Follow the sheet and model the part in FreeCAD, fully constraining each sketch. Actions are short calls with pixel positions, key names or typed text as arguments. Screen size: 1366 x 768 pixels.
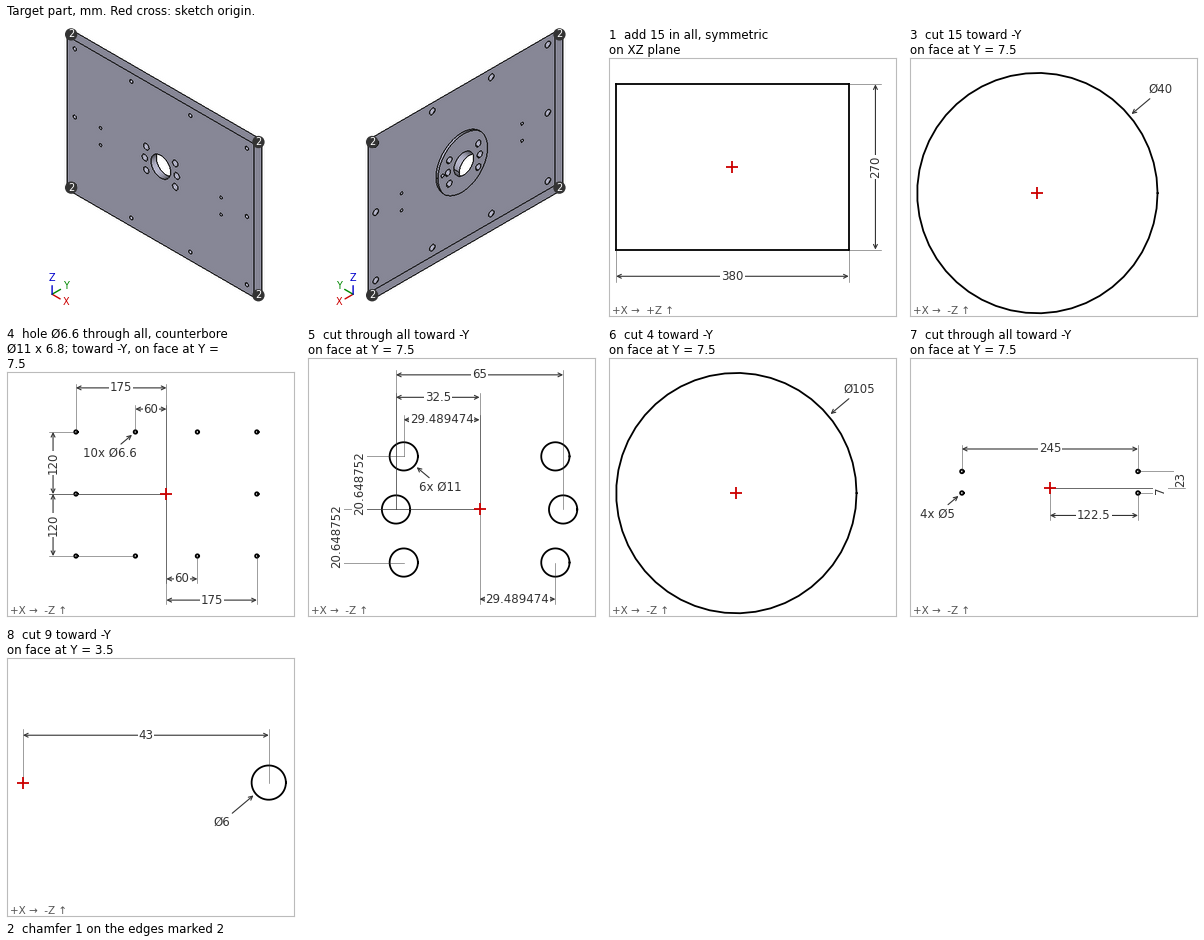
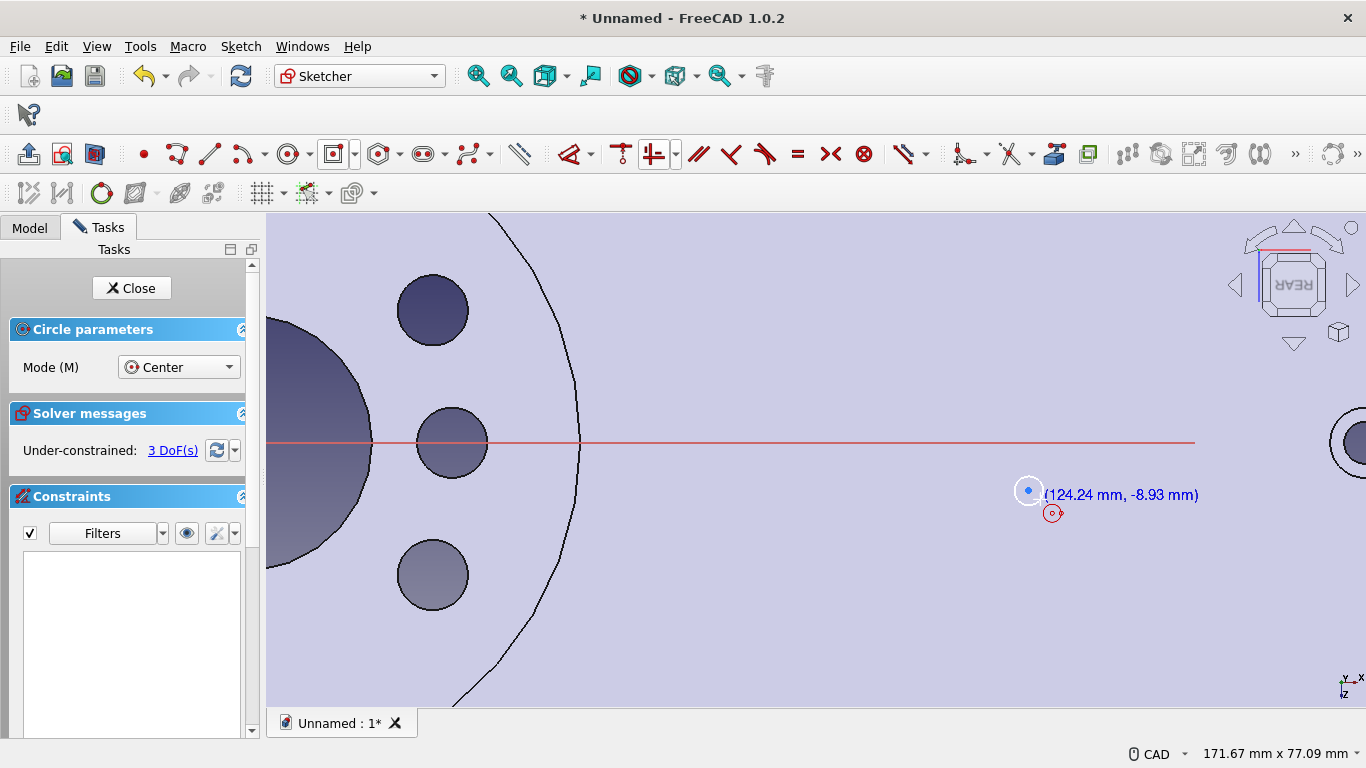
scroll(1029, 295, up, 2)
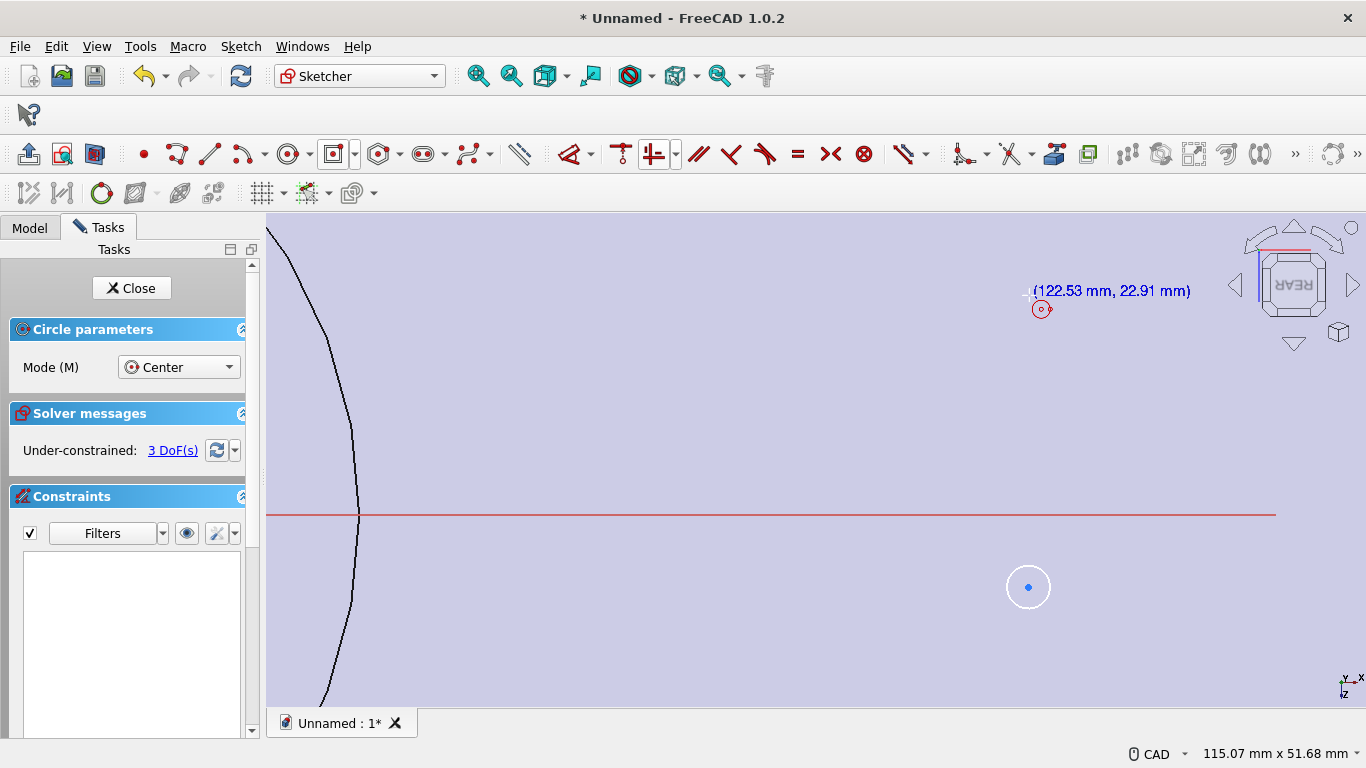
scroll(1039, 467, down, 7)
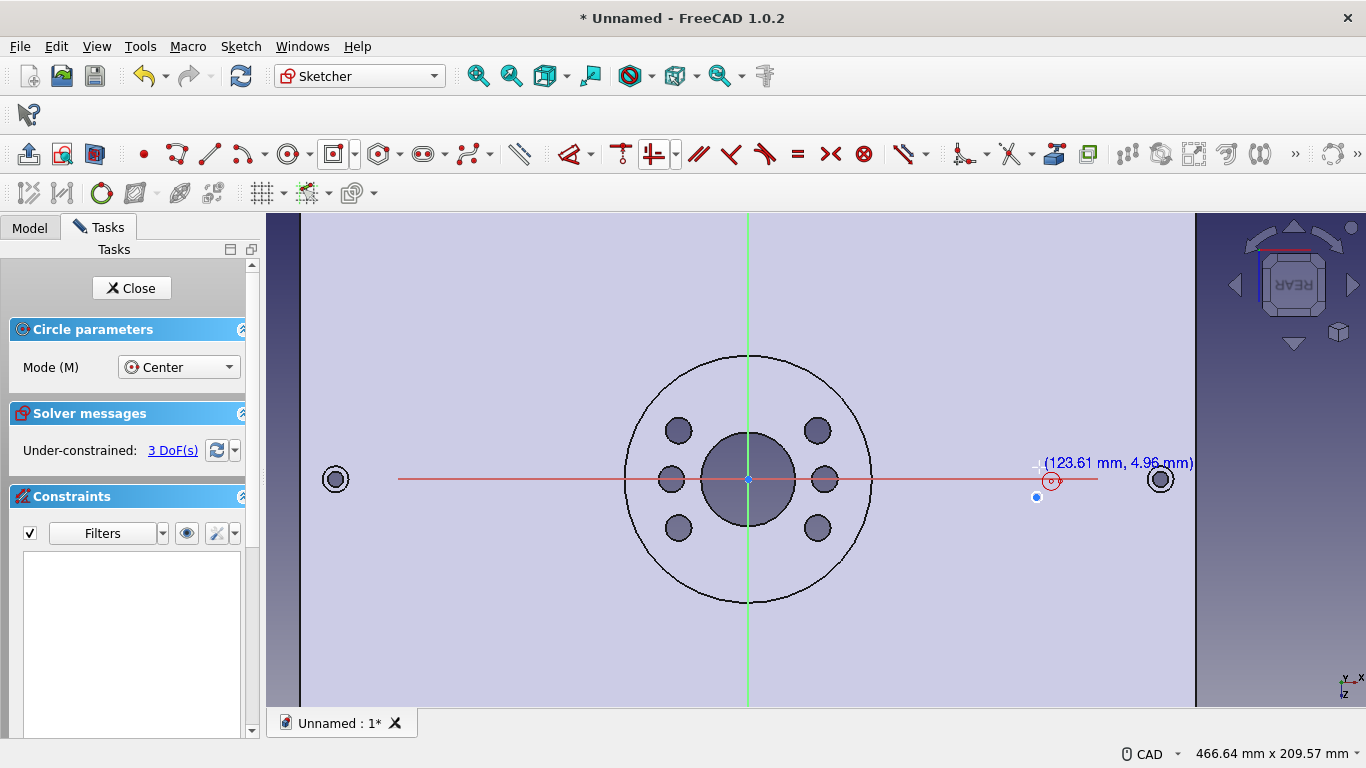
click(1037, 425)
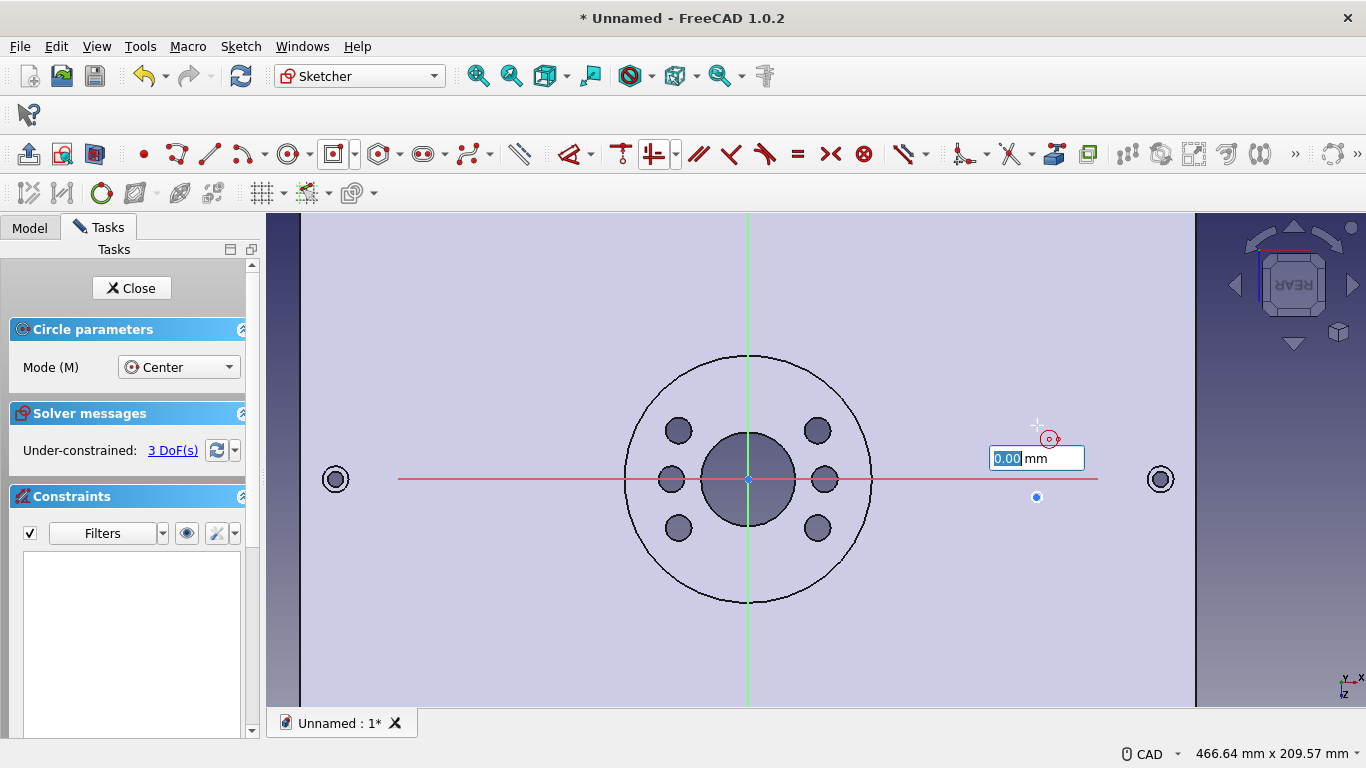
scroll(1041, 421, up, 5)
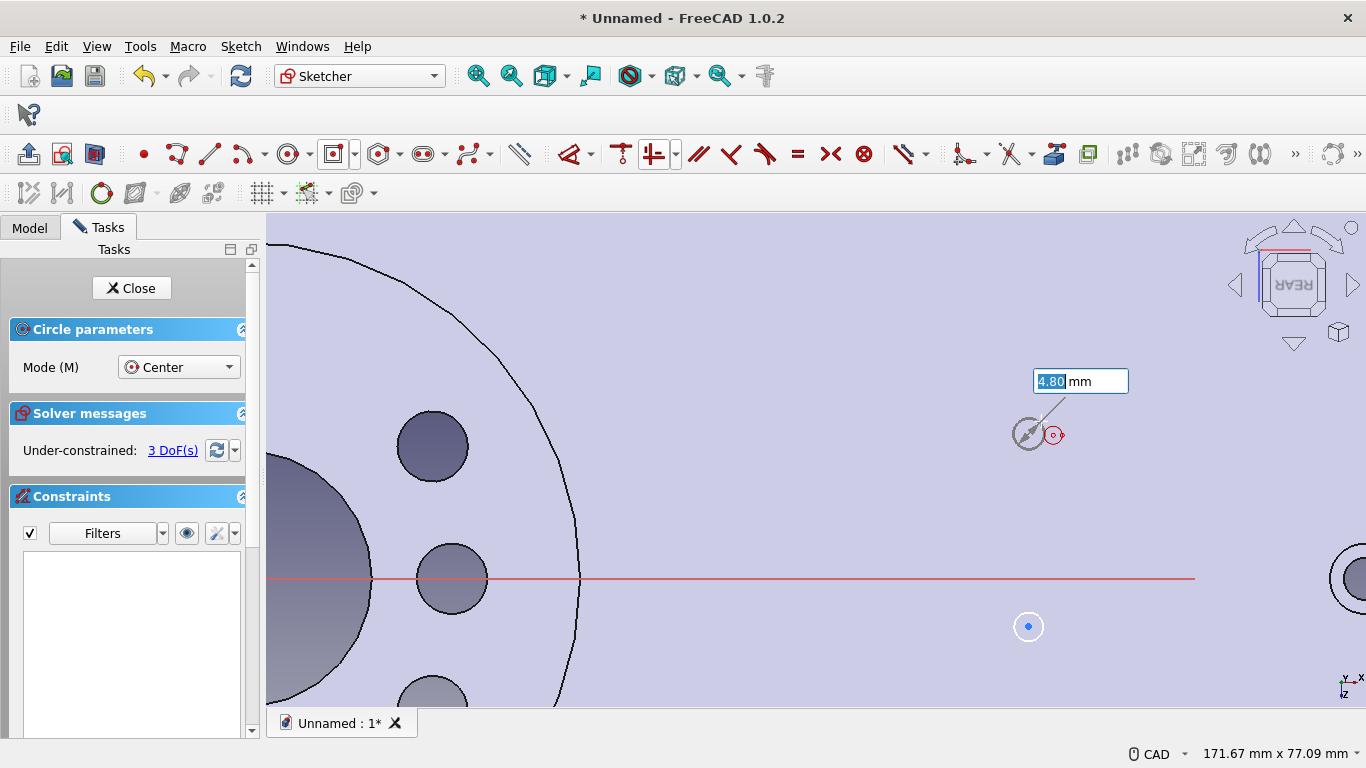
click(1040, 420)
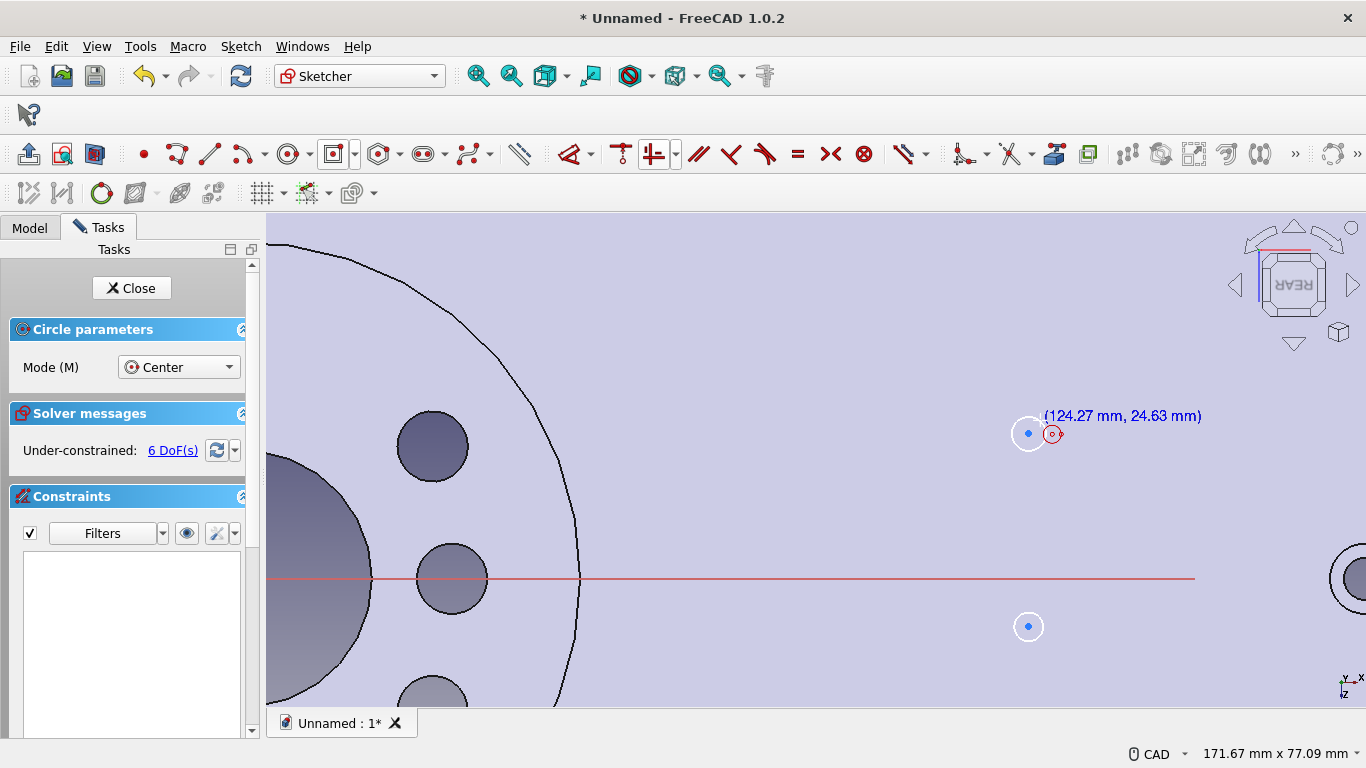
scroll(1041, 421, down, 5)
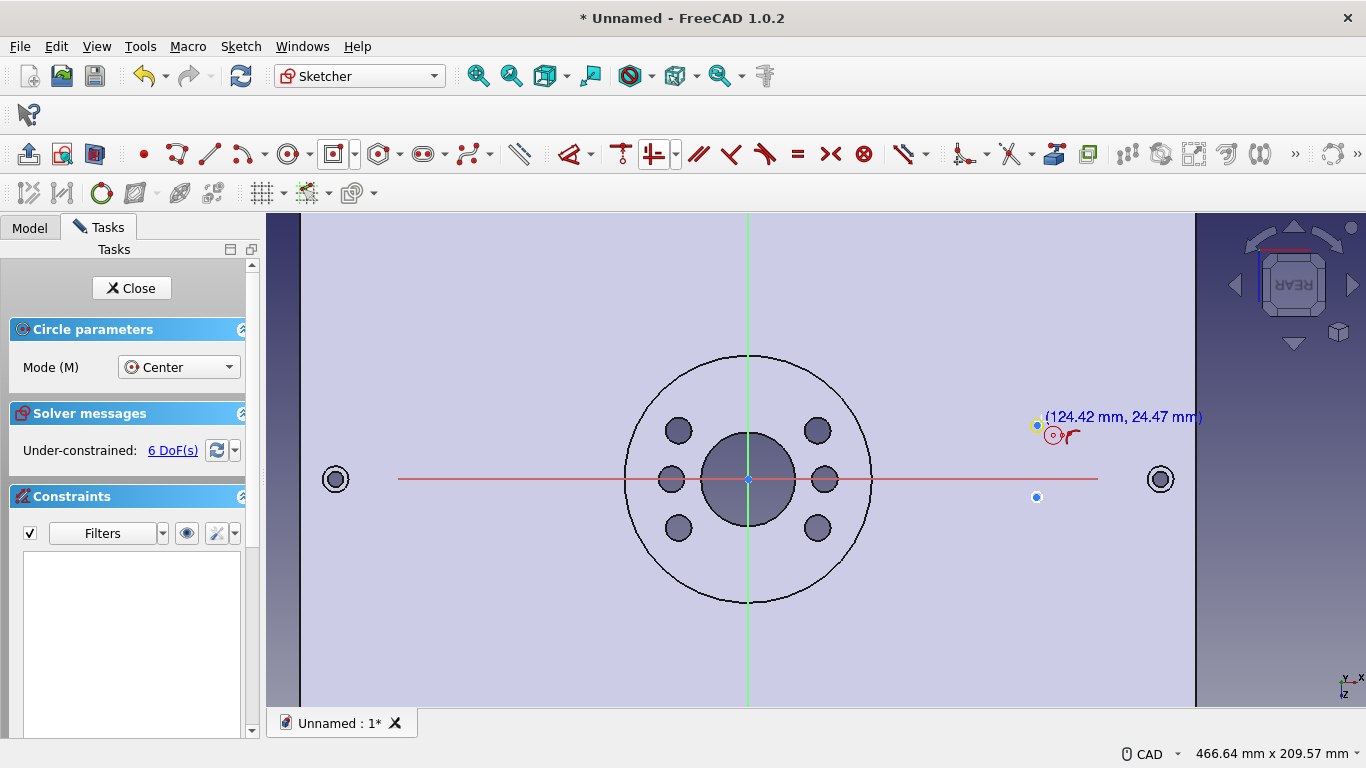
scroll(459, 425, up, 7)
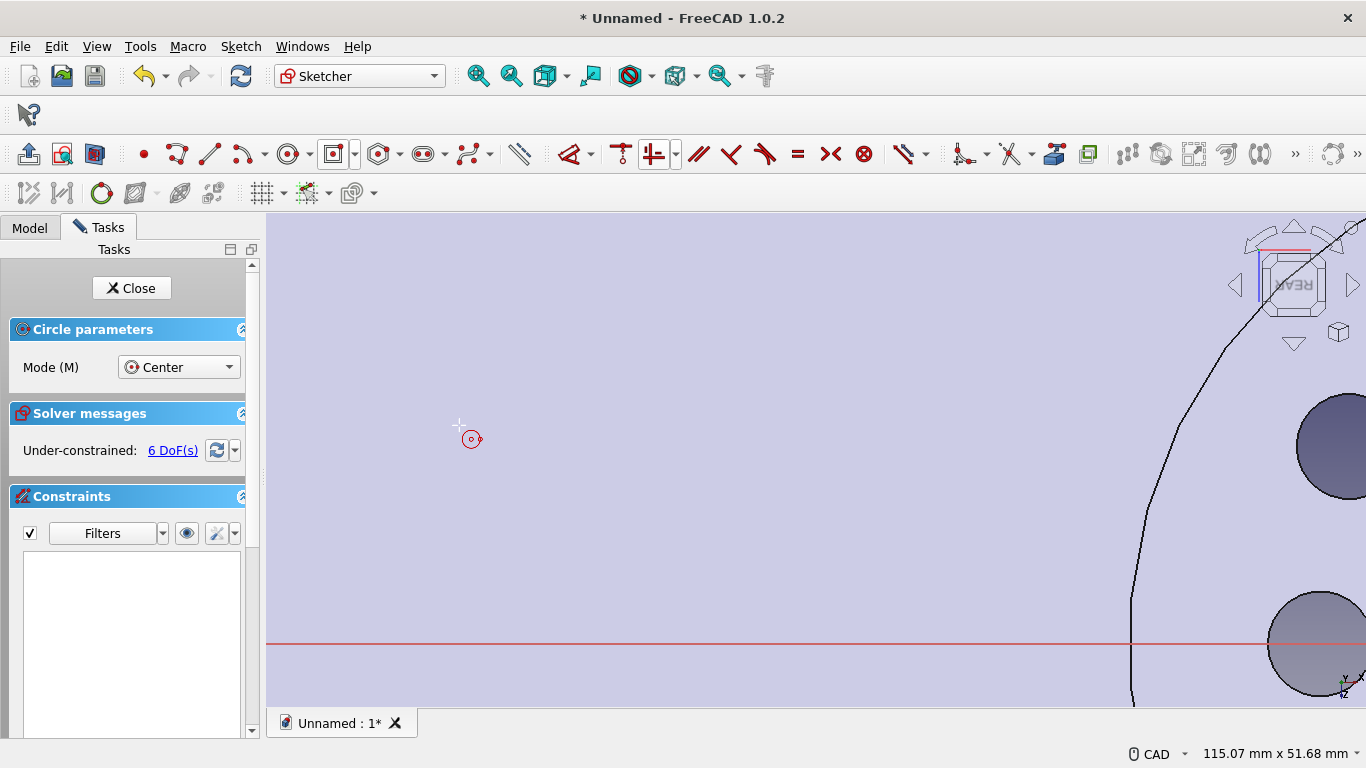
scroll(458, 425, down, 7)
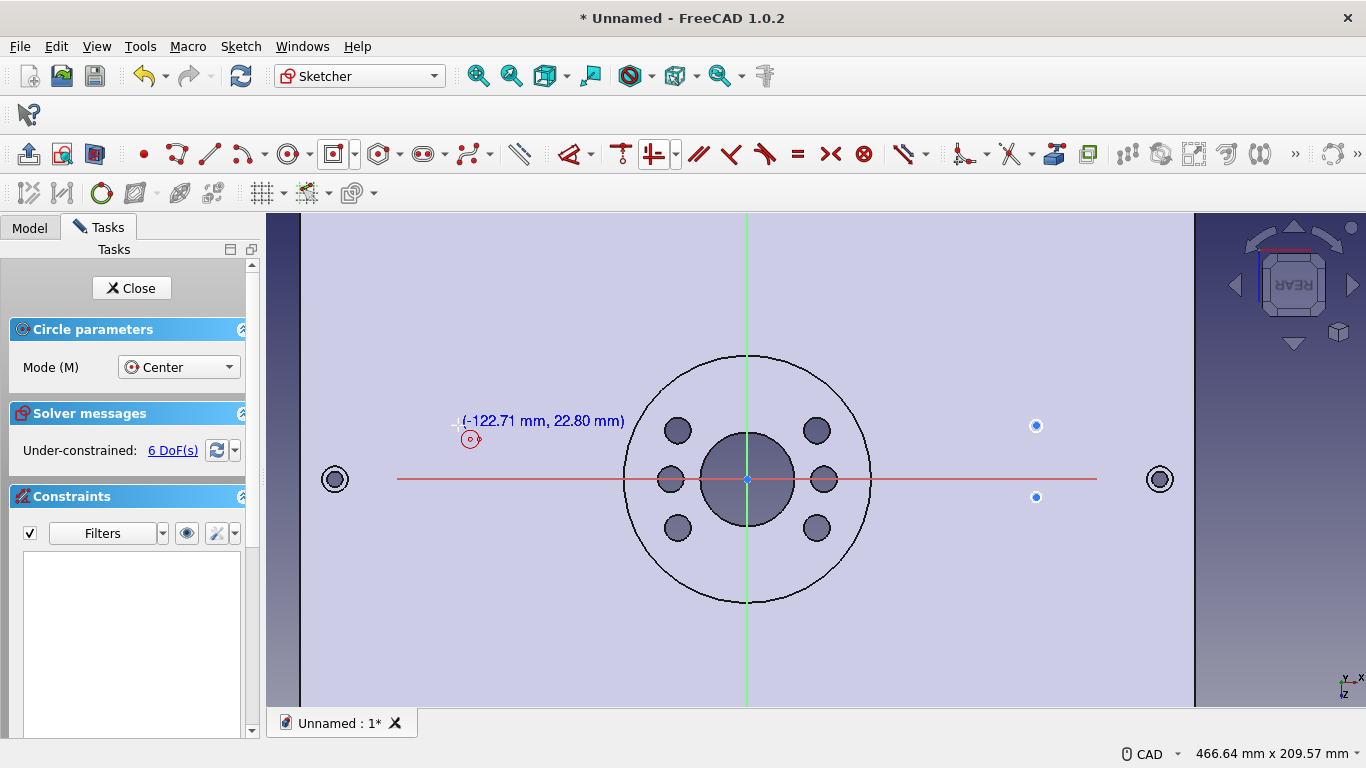
click(459, 425)